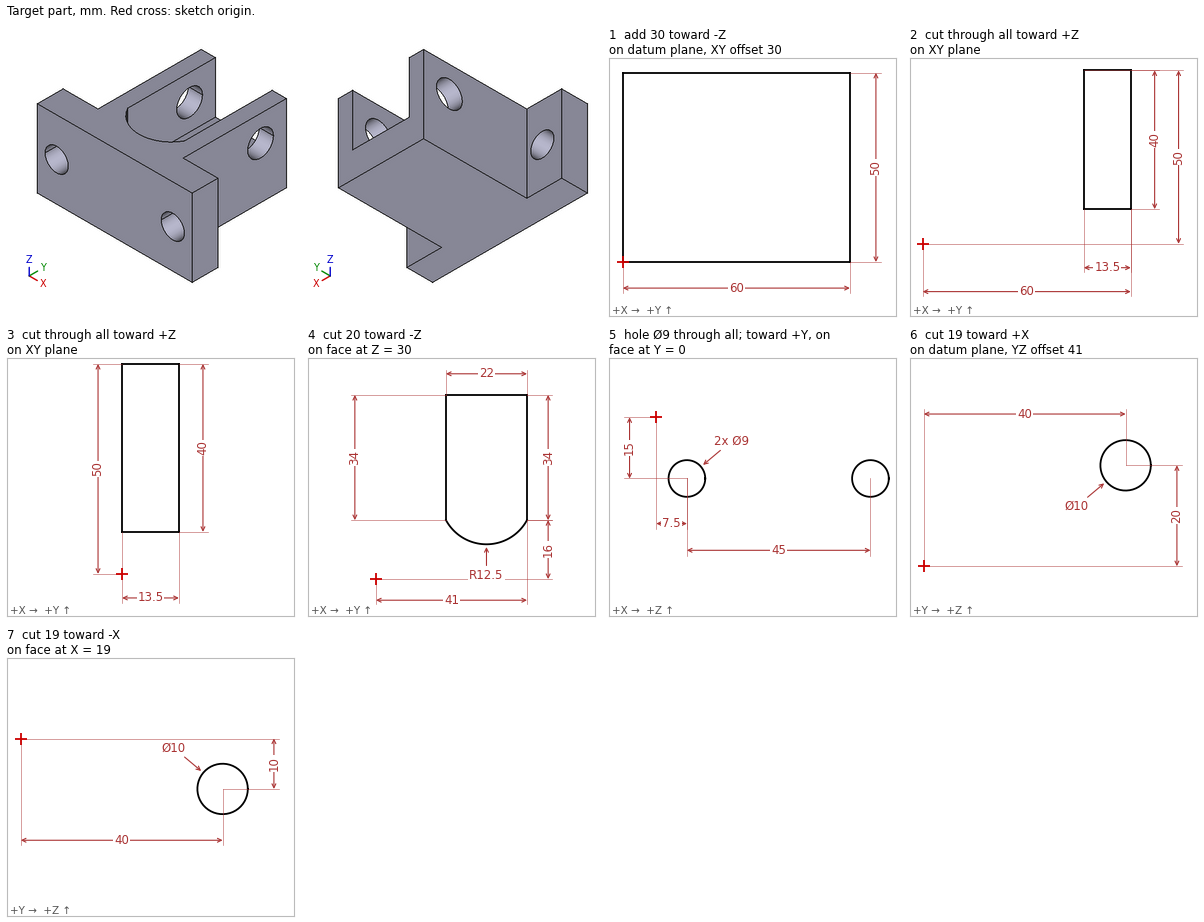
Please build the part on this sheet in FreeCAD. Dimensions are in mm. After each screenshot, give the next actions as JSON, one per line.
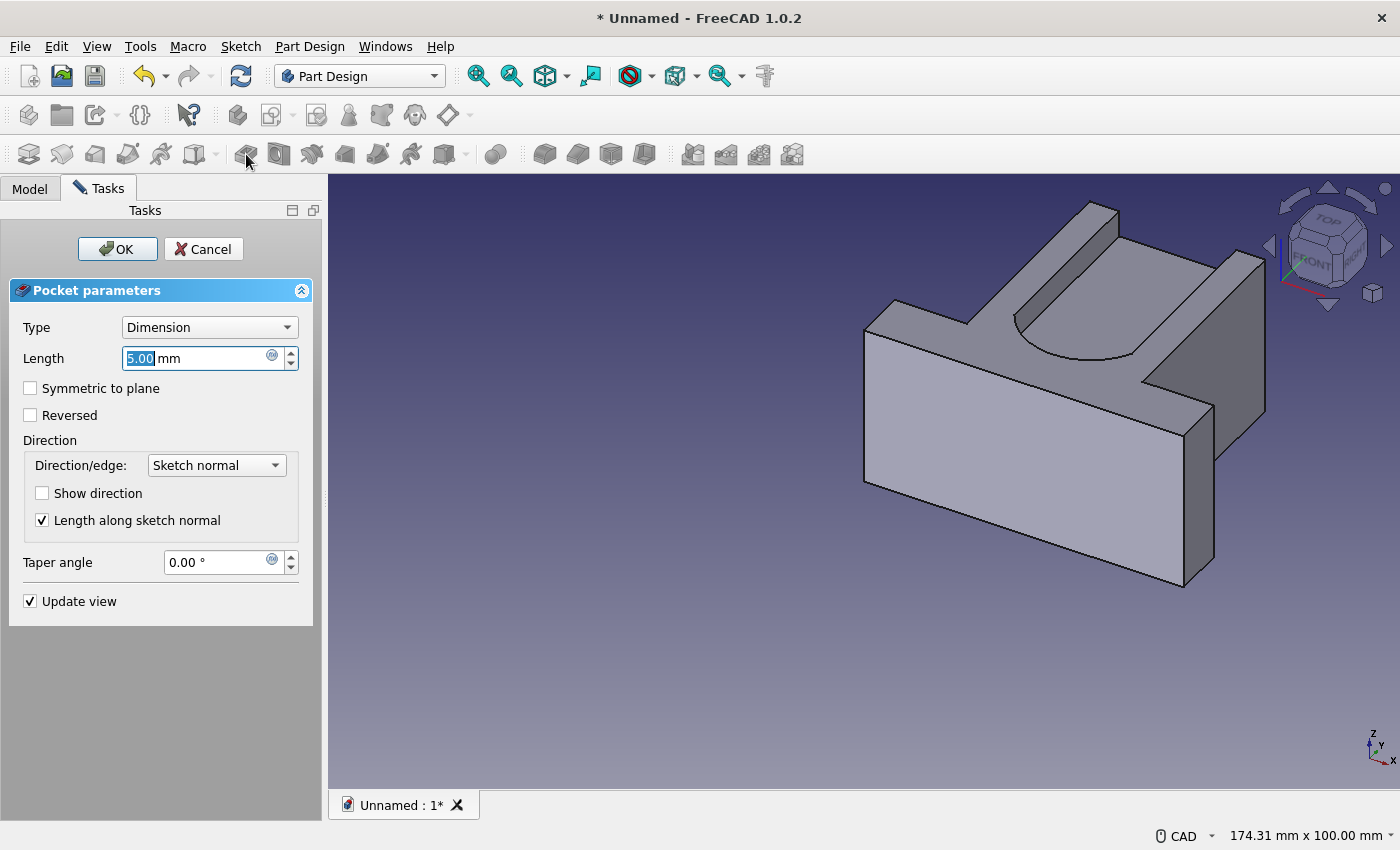
{"action": "type", "text": "20"}
{"action": "key", "text": "Tab"}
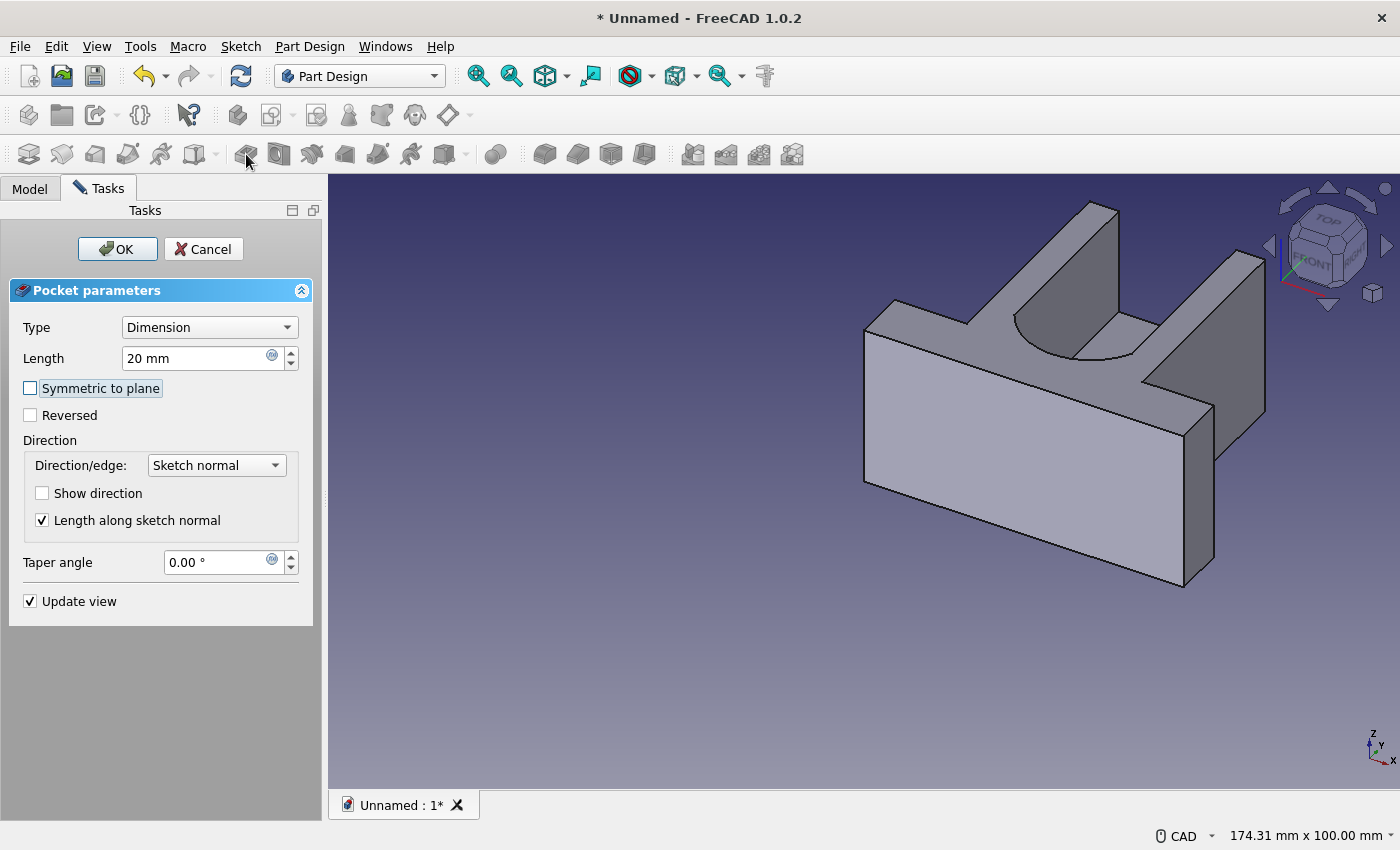
{"action": "left_click", "coordinate": [118, 249]}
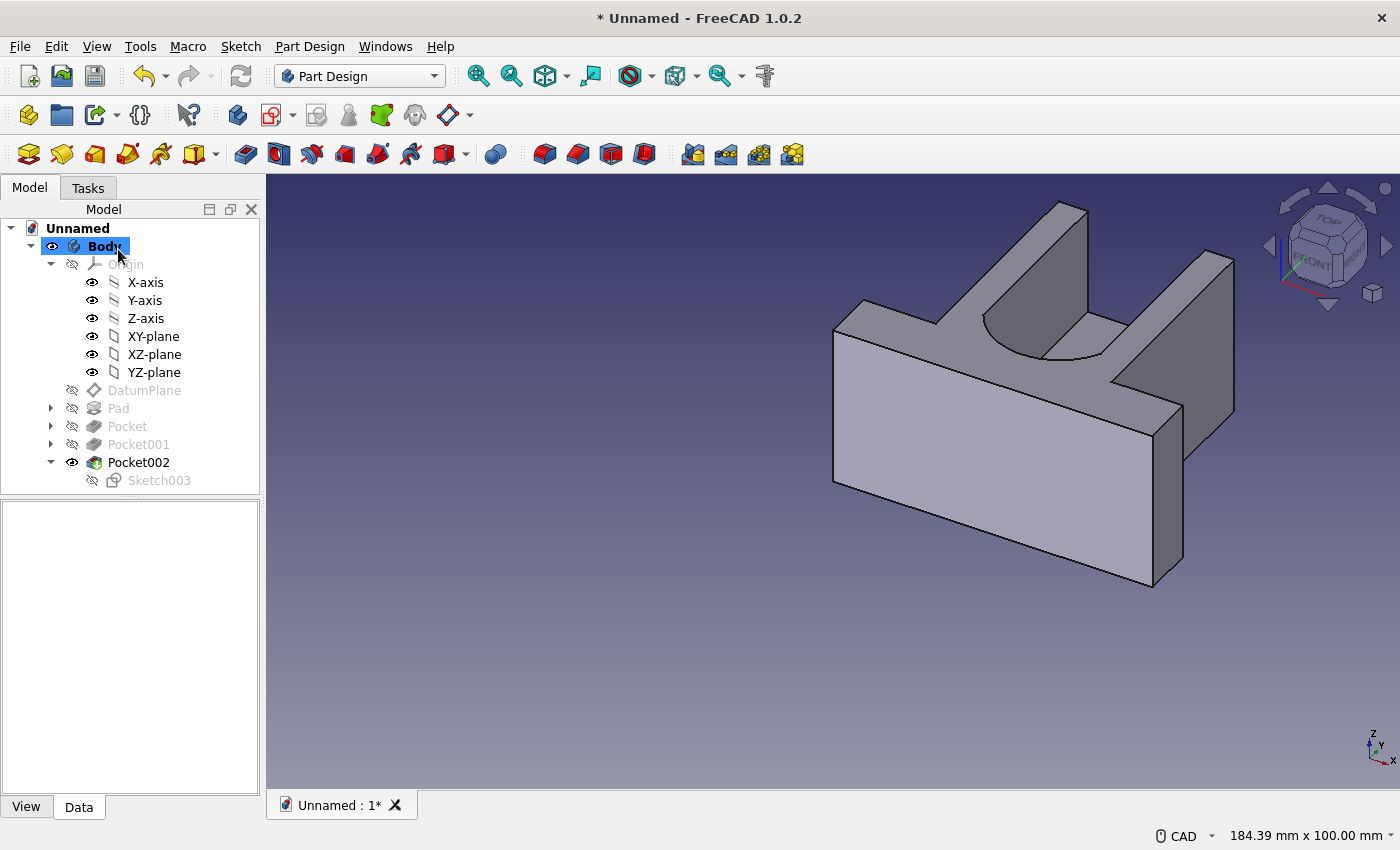
{"action": "left_click", "coordinate": [1038, 473]}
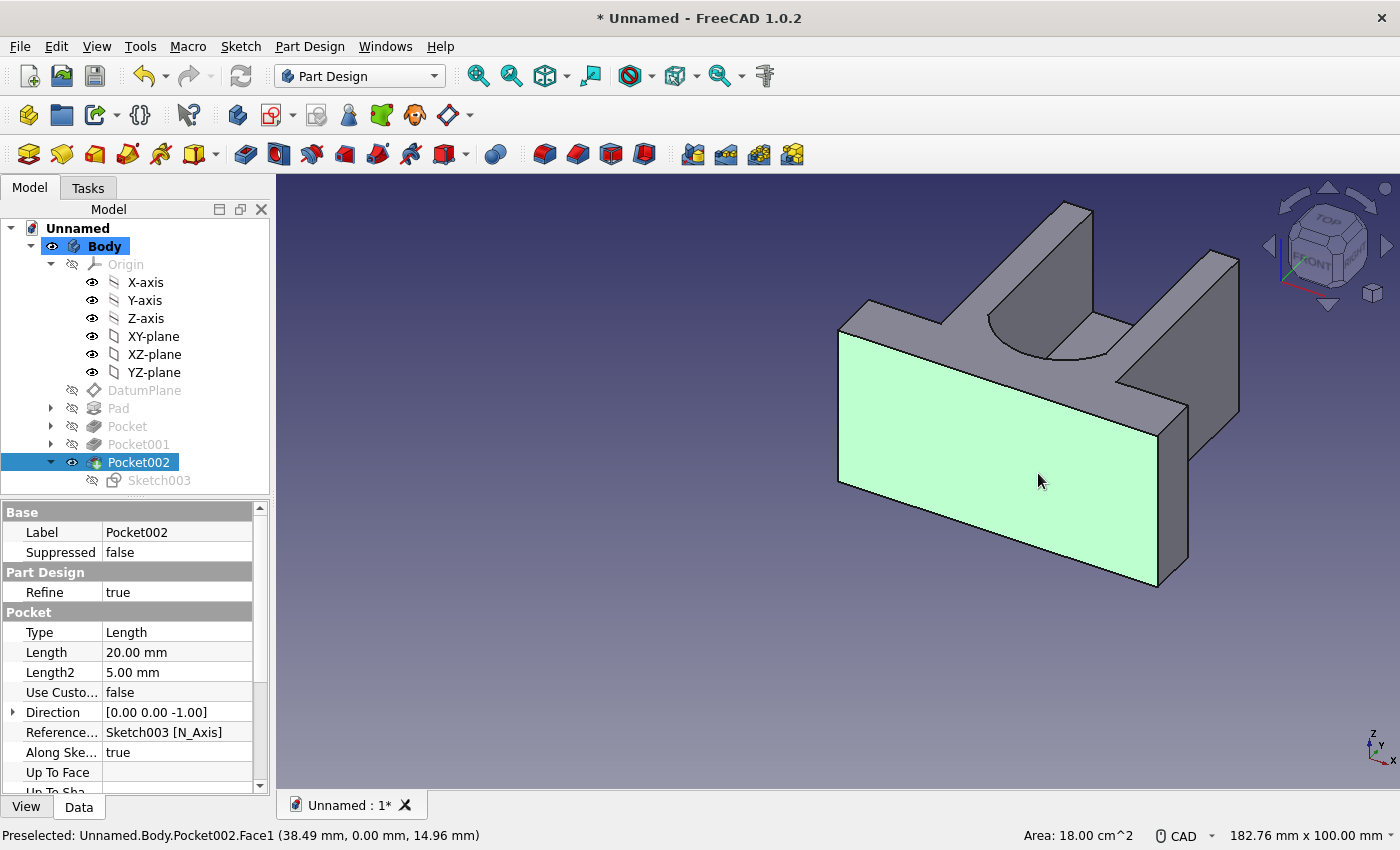
{"action": "left_click", "coordinate": [270, 116]}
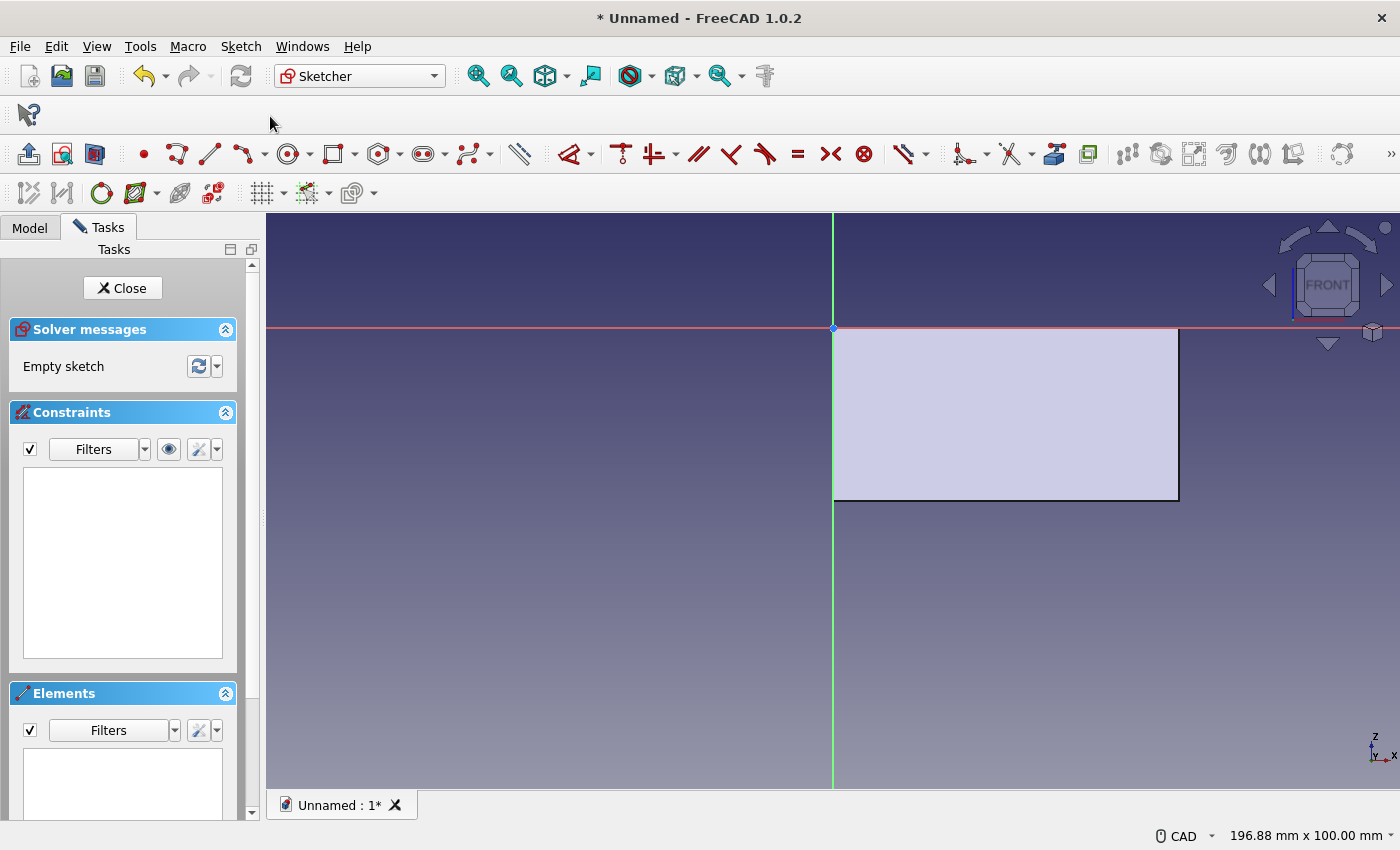
{"action": "scroll", "coordinate": [1187, 289], "scroll_direction": "up", "scroll_amount": 4}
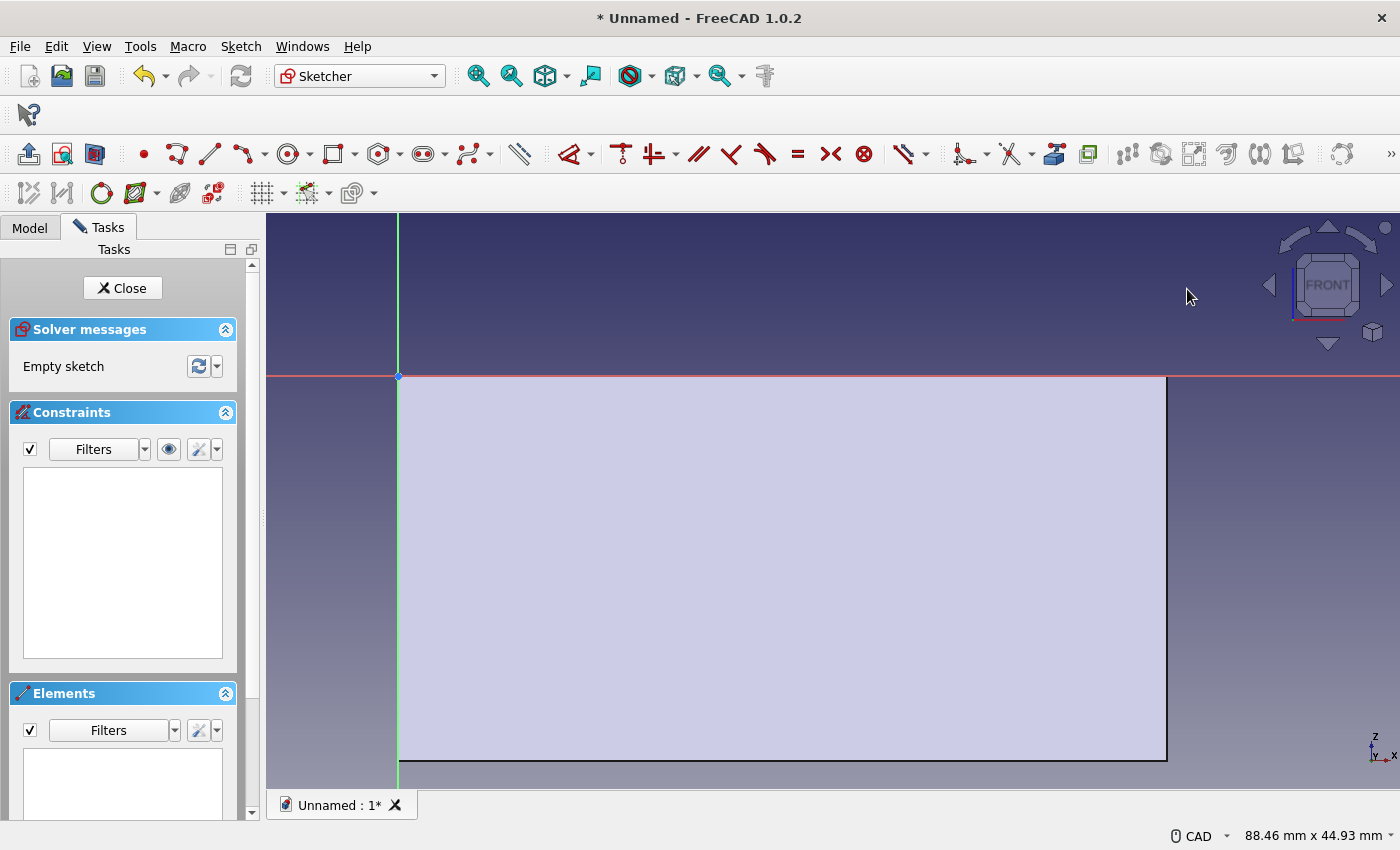
{"action": "key", "text": "g c"}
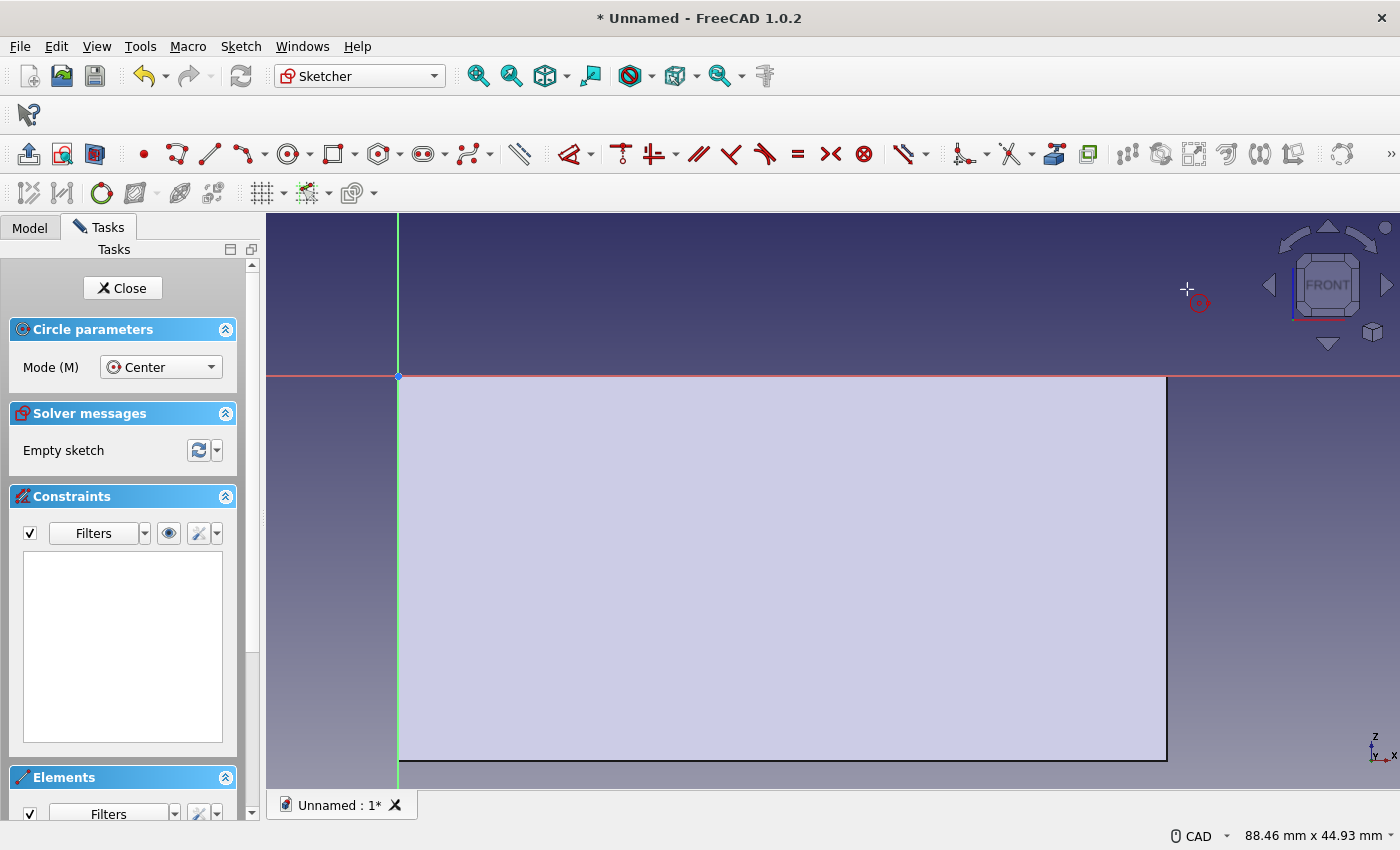
{"action": "left_click", "coordinate": [494, 568]}
{"action": "mouse_move", "coordinate": [535, 528]}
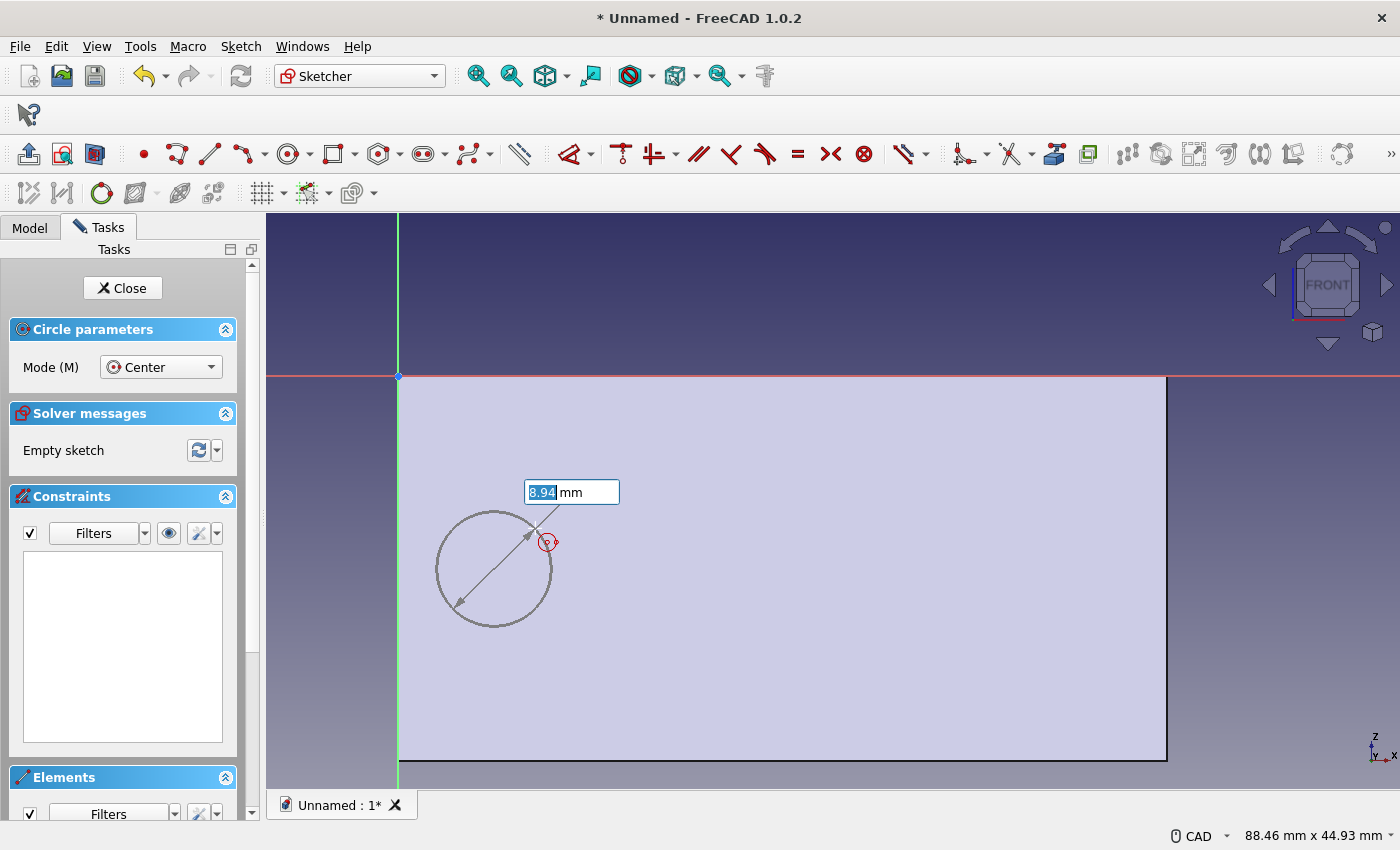
{"action": "type", "text": "9"}
{"action": "key", "text": "Return"}